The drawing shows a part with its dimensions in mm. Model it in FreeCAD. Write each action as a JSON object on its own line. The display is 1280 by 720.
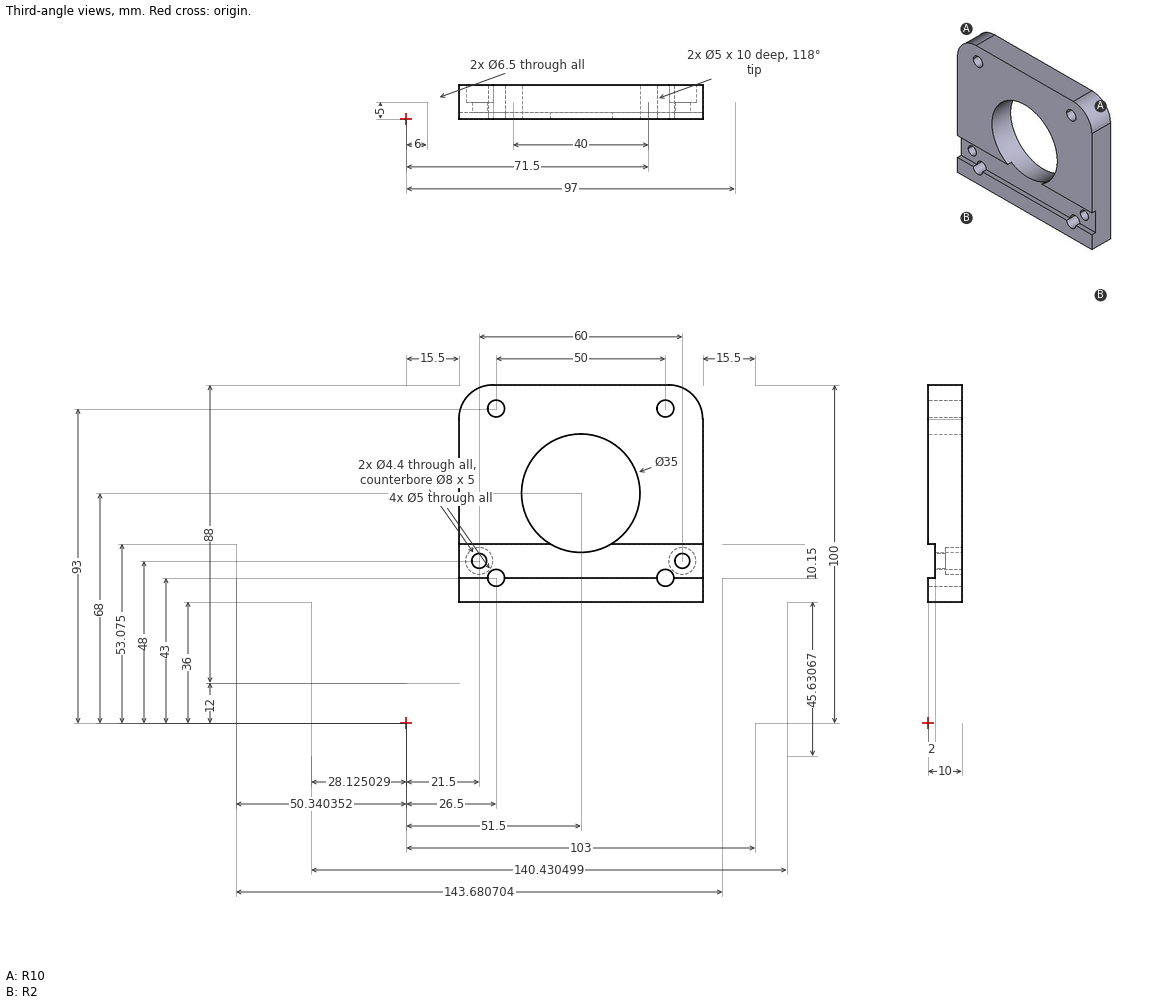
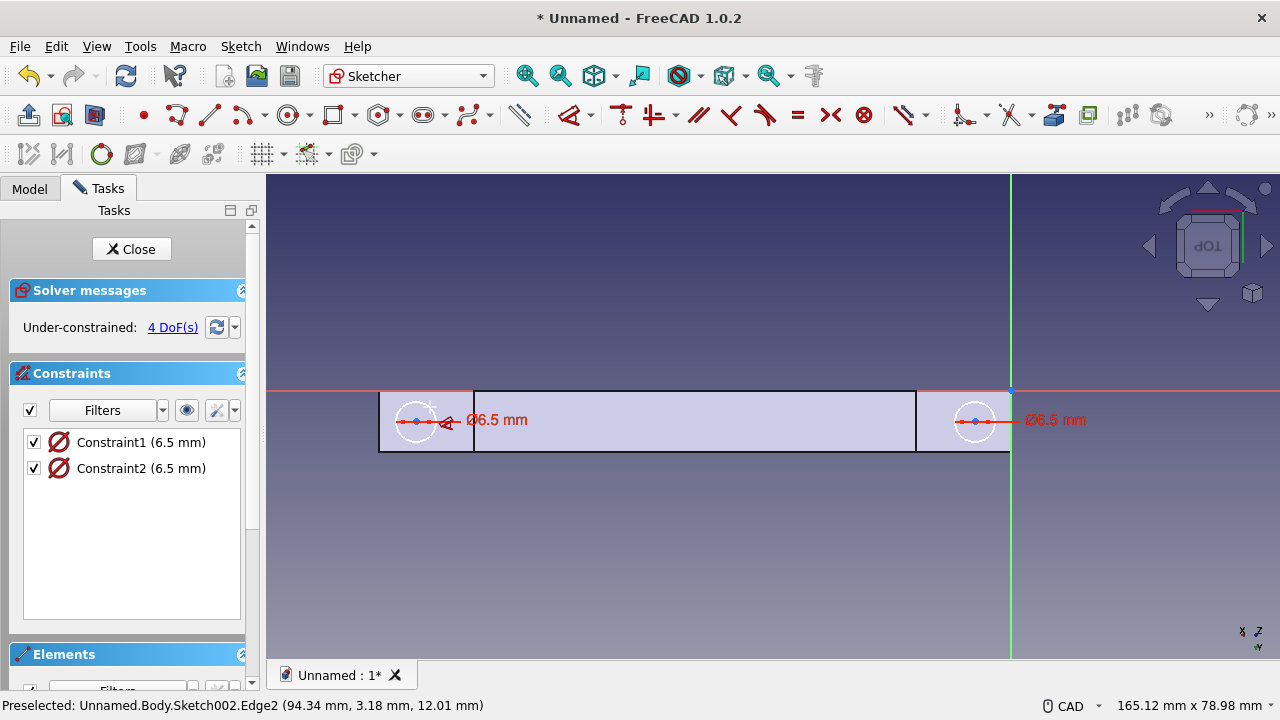
{"action": "left_click", "coordinate": [975, 422]}
{"action": "left_click", "coordinate": [993, 357]}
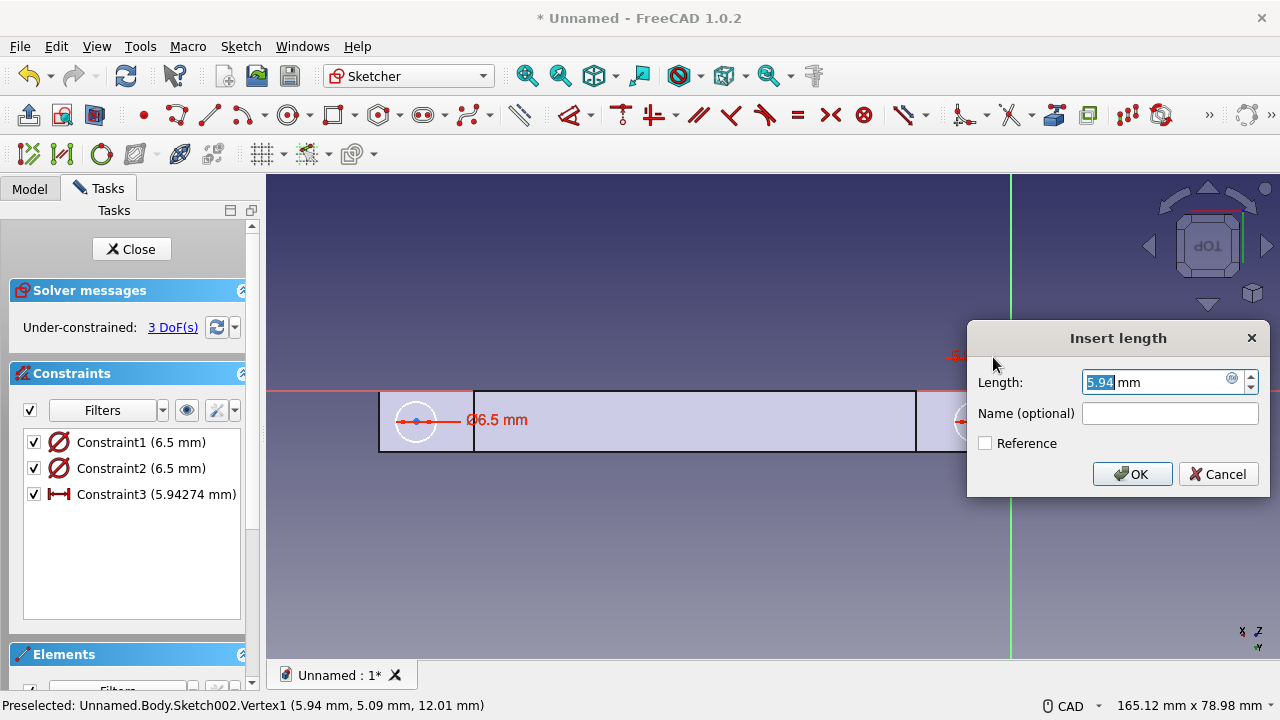
{"action": "type", "text": "6"}
{"action": "key", "text": "Return"}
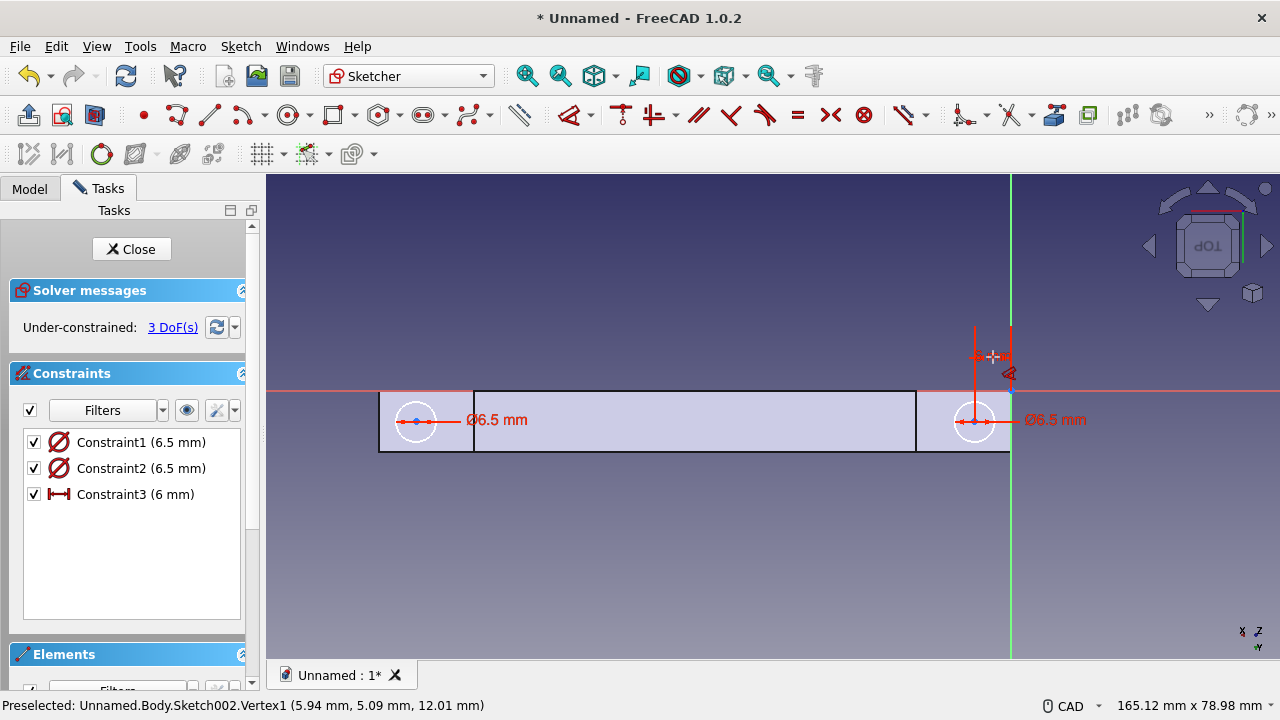
{"action": "scroll", "coordinate": [975, 422], "scroll_direction": "up", "scroll_amount": 2}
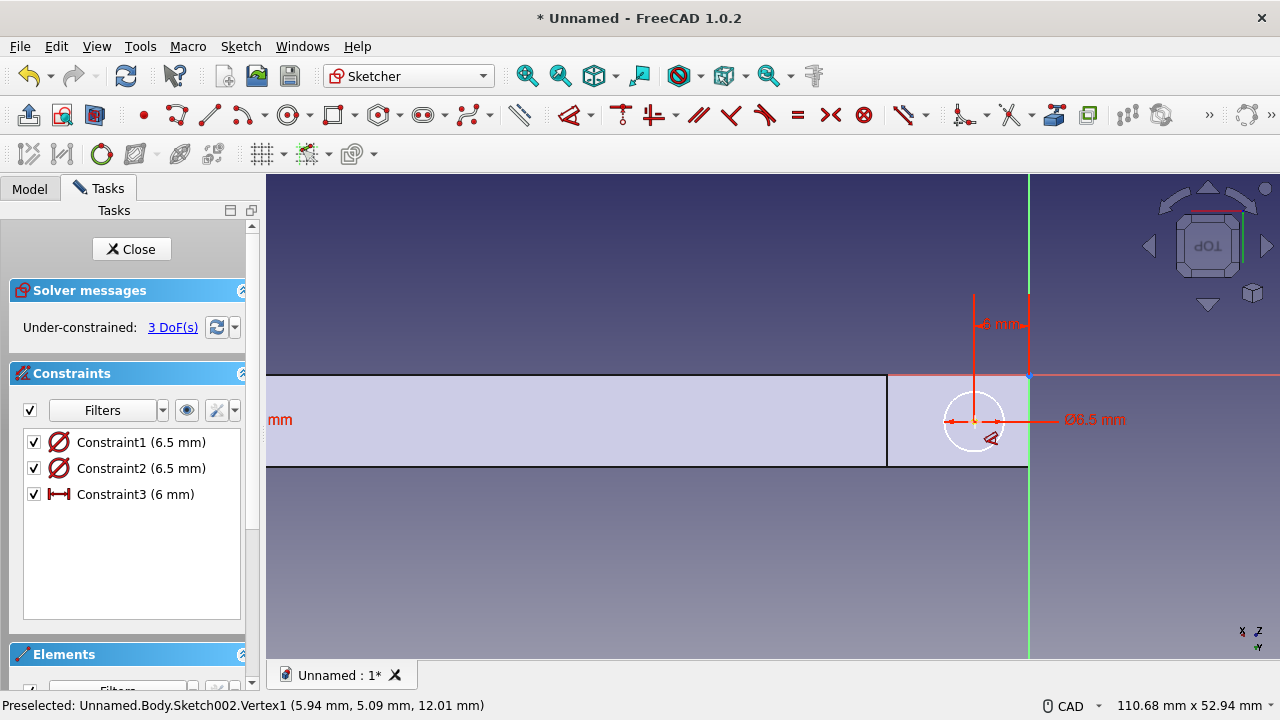
{"action": "left_click", "coordinate": [974, 422]}
{"action": "left_click", "coordinate": [1063, 398]}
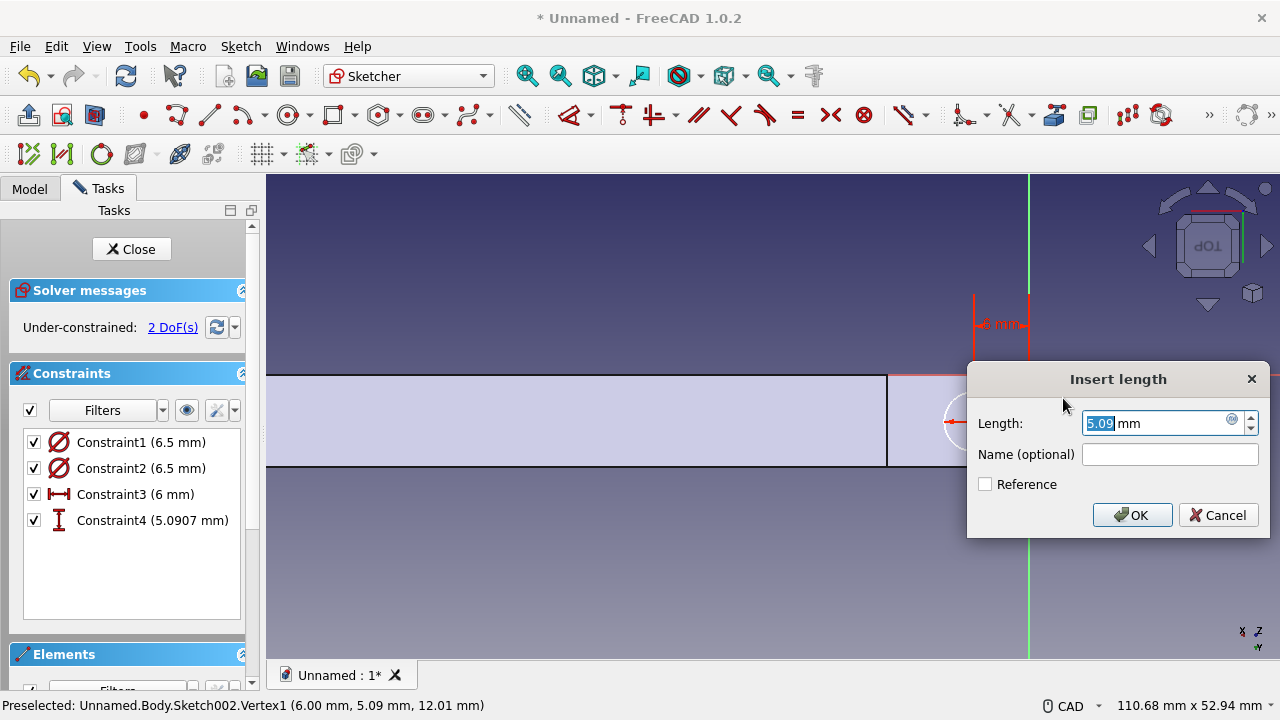
{"action": "type", "text": "5"}
{"action": "key", "text": "Return"}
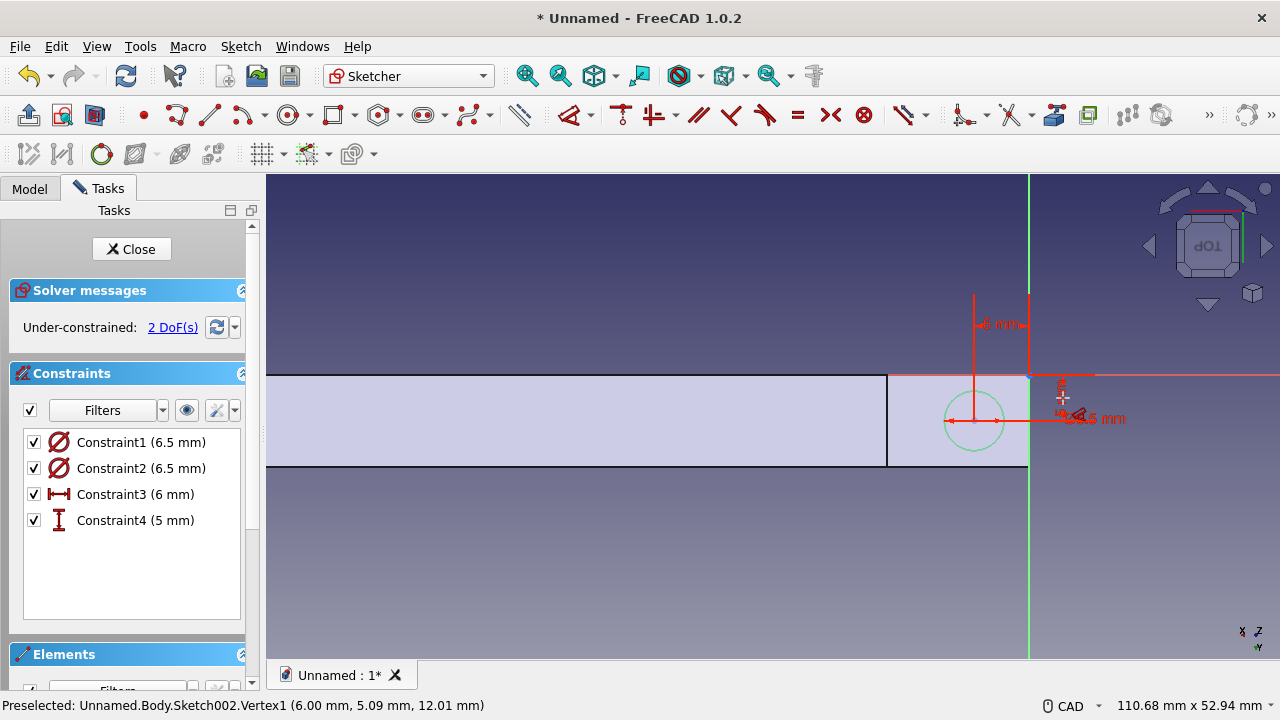
{"action": "scroll", "coordinate": [978, 424], "scroll_direction": "down", "scroll_amount": 2}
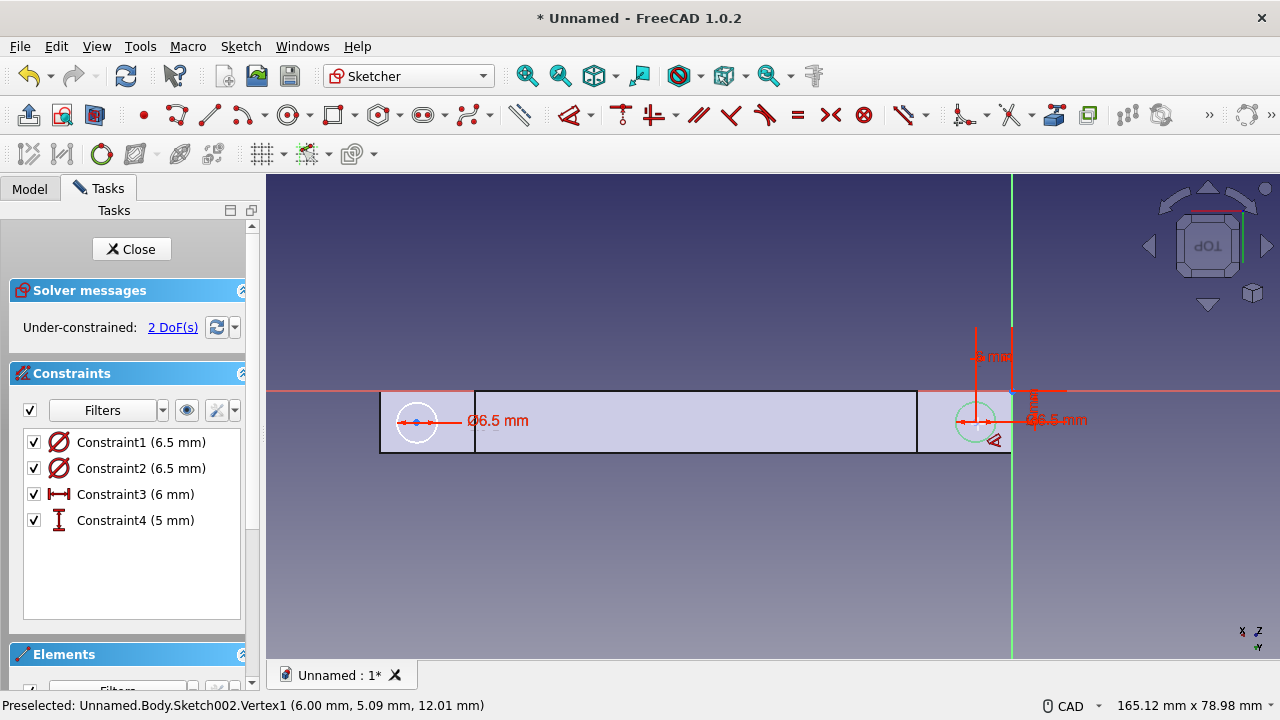
{"action": "scroll", "coordinate": [417, 423], "scroll_direction": "up", "scroll_amount": 2}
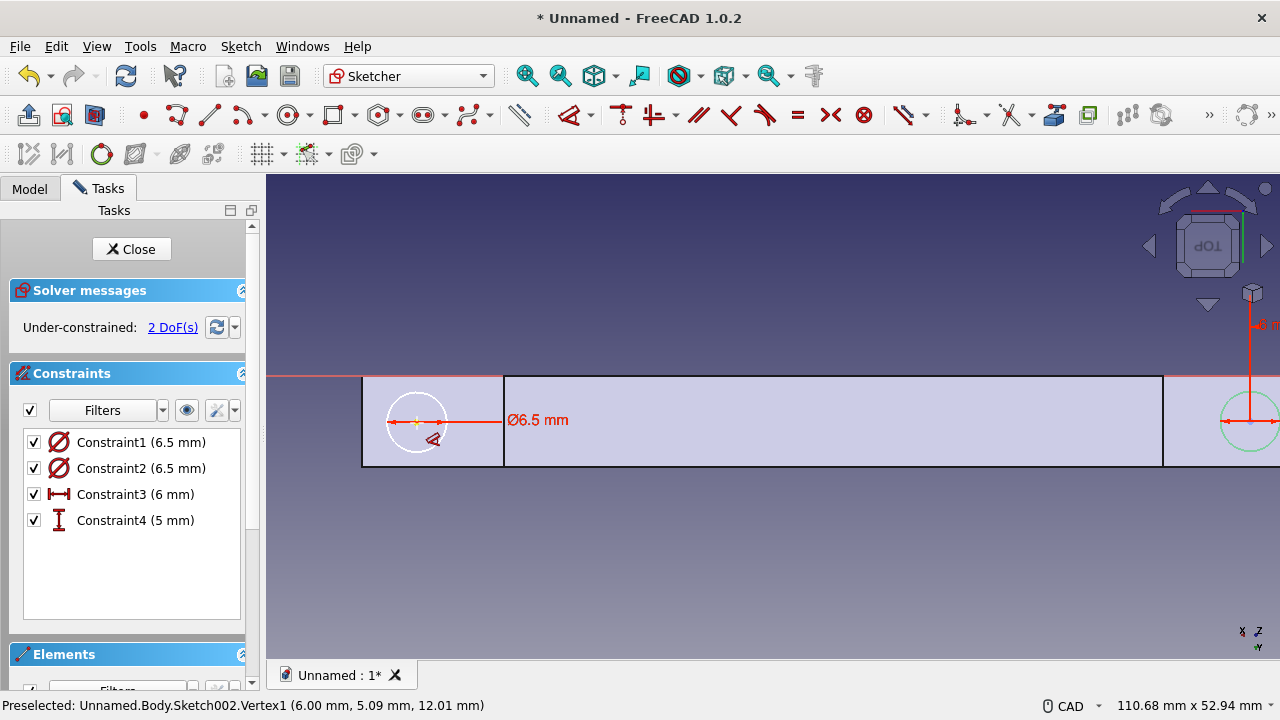
{"action": "left_click", "coordinate": [417, 422]}
{"action": "left_click", "coordinate": [359, 399]}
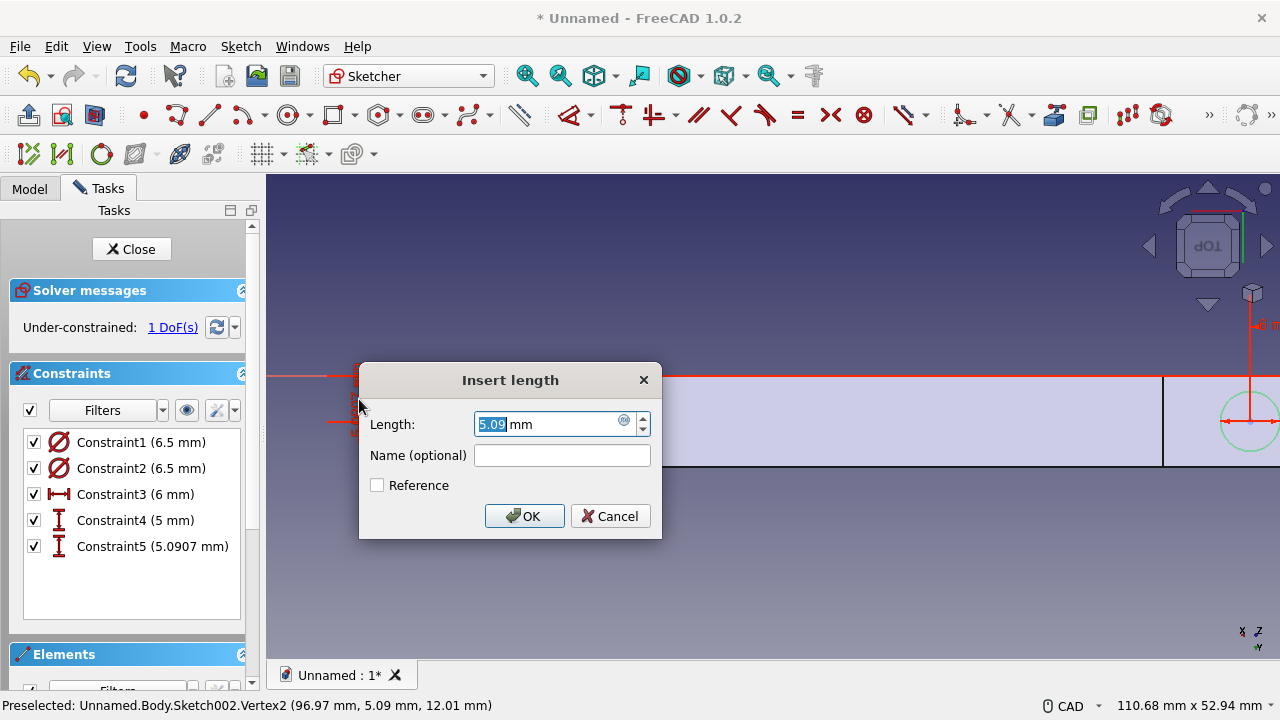
{"action": "type", "text": "5"}
{"action": "key", "text": "Return"}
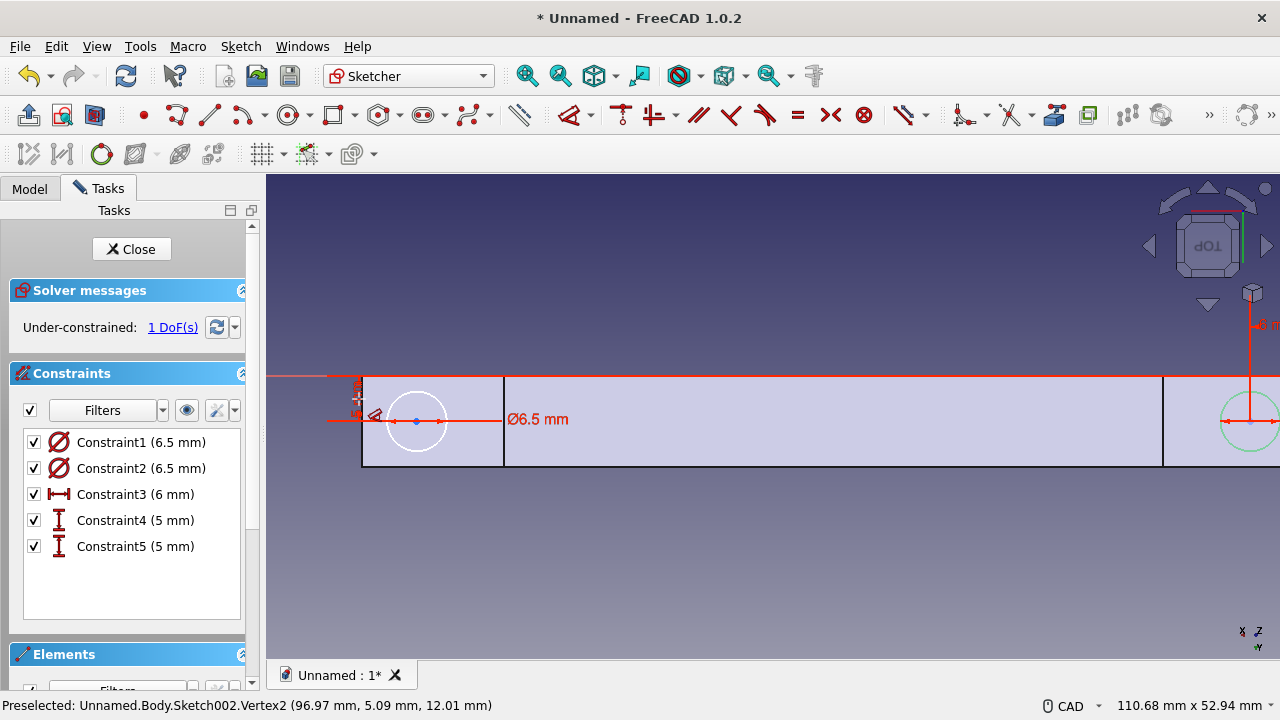
{"action": "left_click", "coordinate": [417, 421]}
{"action": "left_click", "coordinate": [766, 342]}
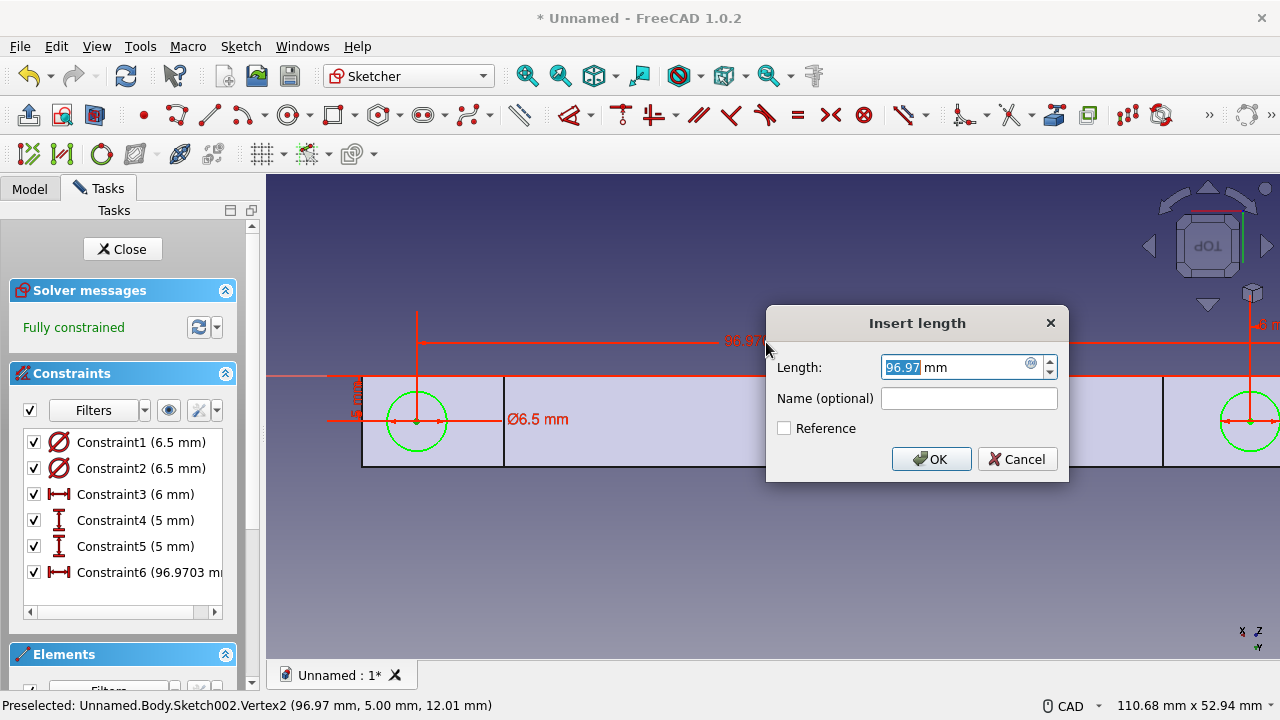
{"action": "type", "text": "97"}
{"action": "key", "text": "Return"}
{"action": "key", "text": "Escape"}